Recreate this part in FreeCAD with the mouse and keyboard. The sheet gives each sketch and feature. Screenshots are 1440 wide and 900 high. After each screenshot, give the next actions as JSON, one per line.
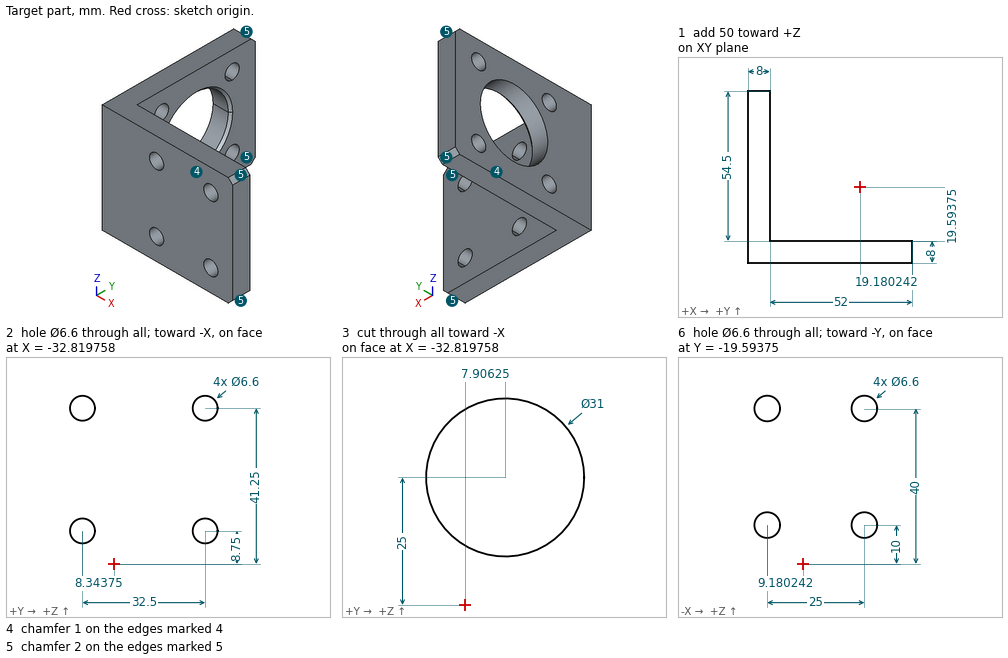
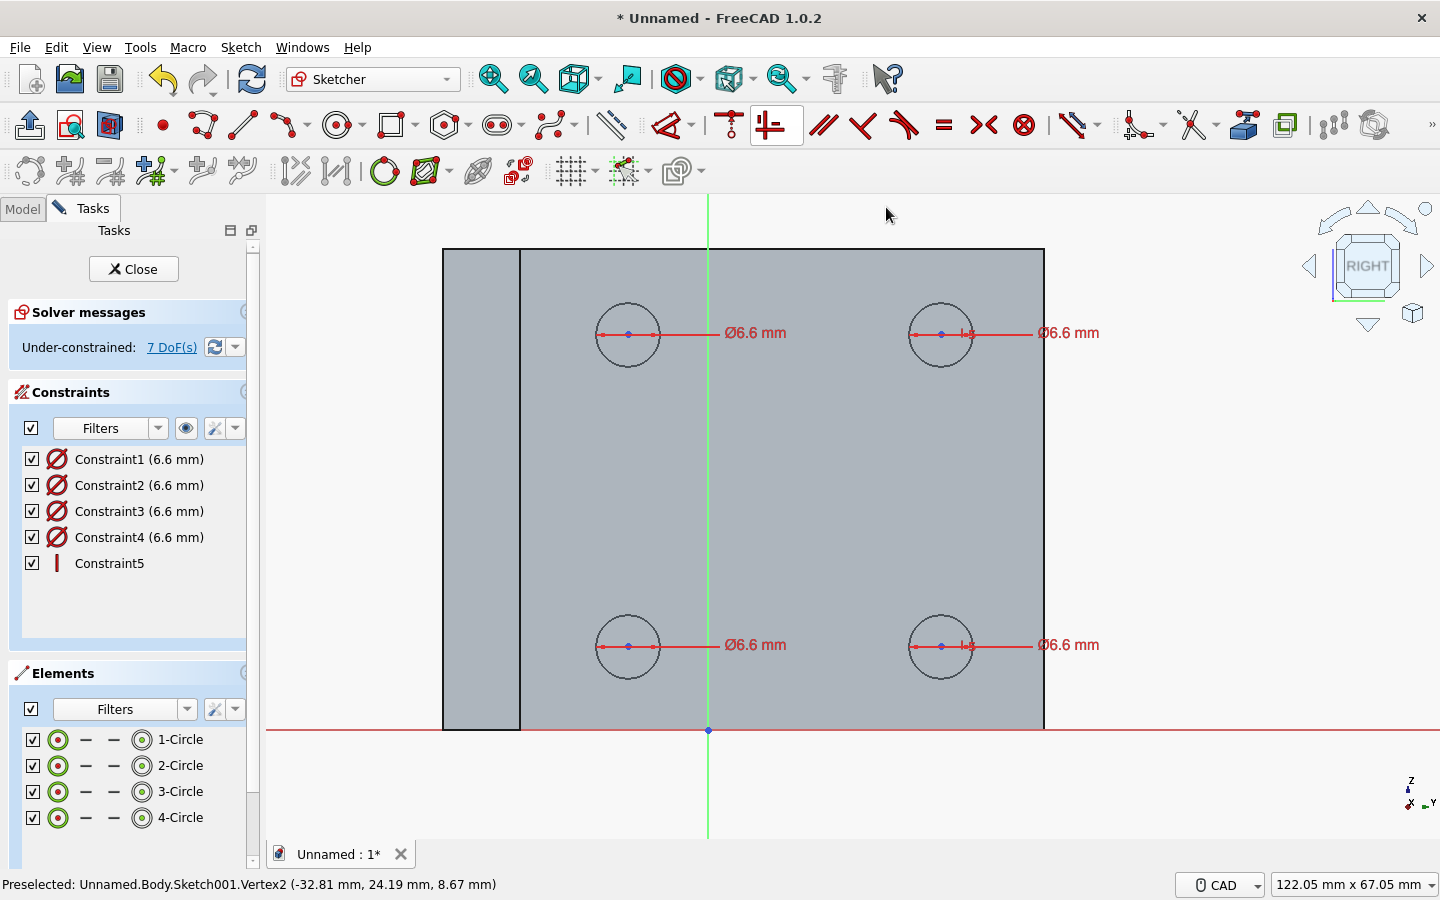
{"action": "left_click", "coordinate": [941, 647]}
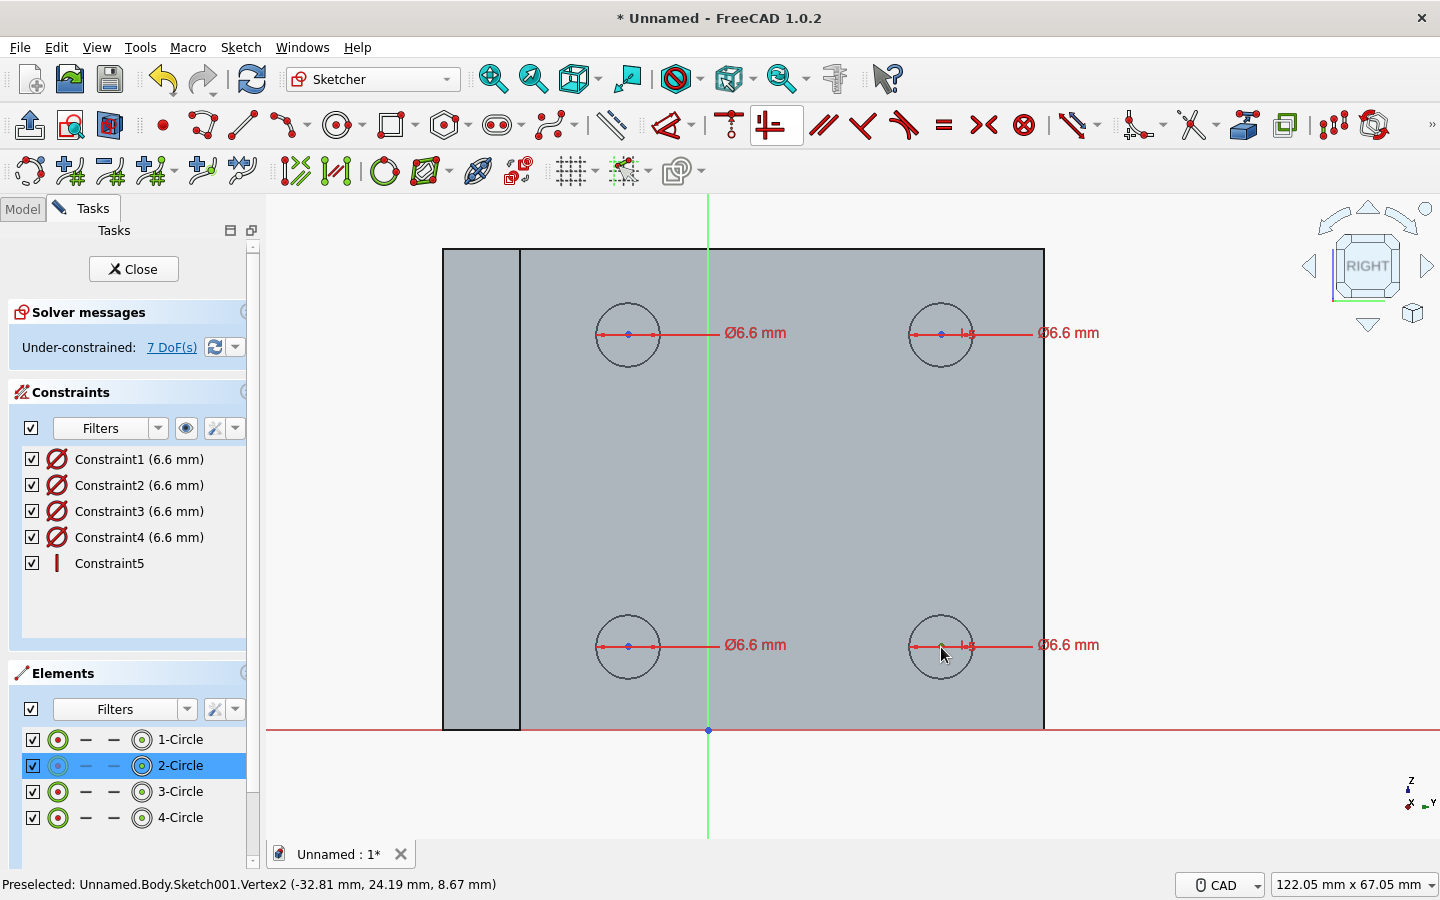
{"action": "left_click", "coordinate": [628, 647]}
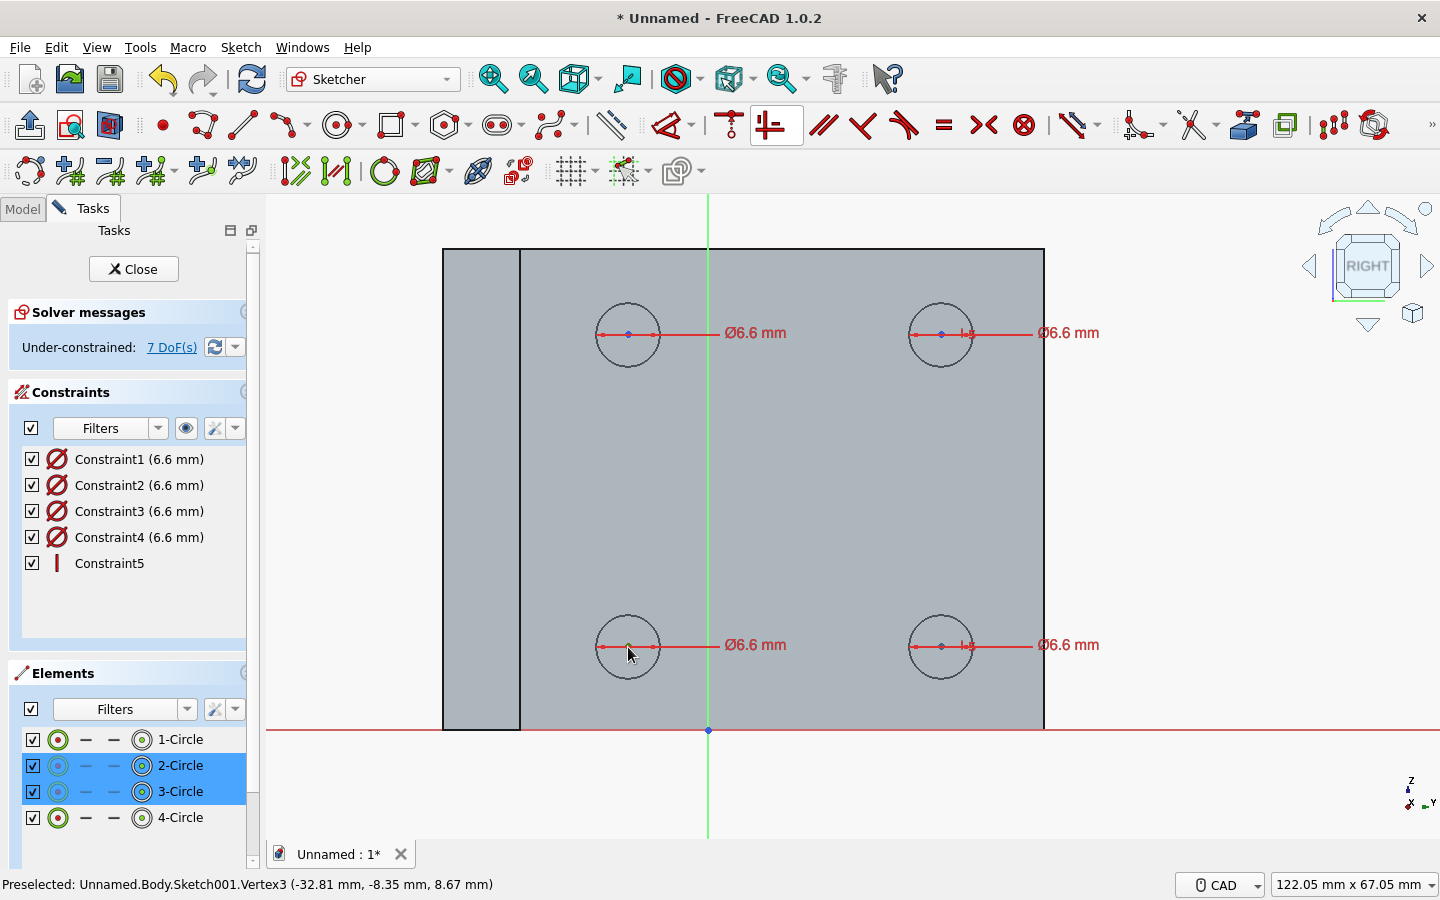
{"action": "key", "text": "h"}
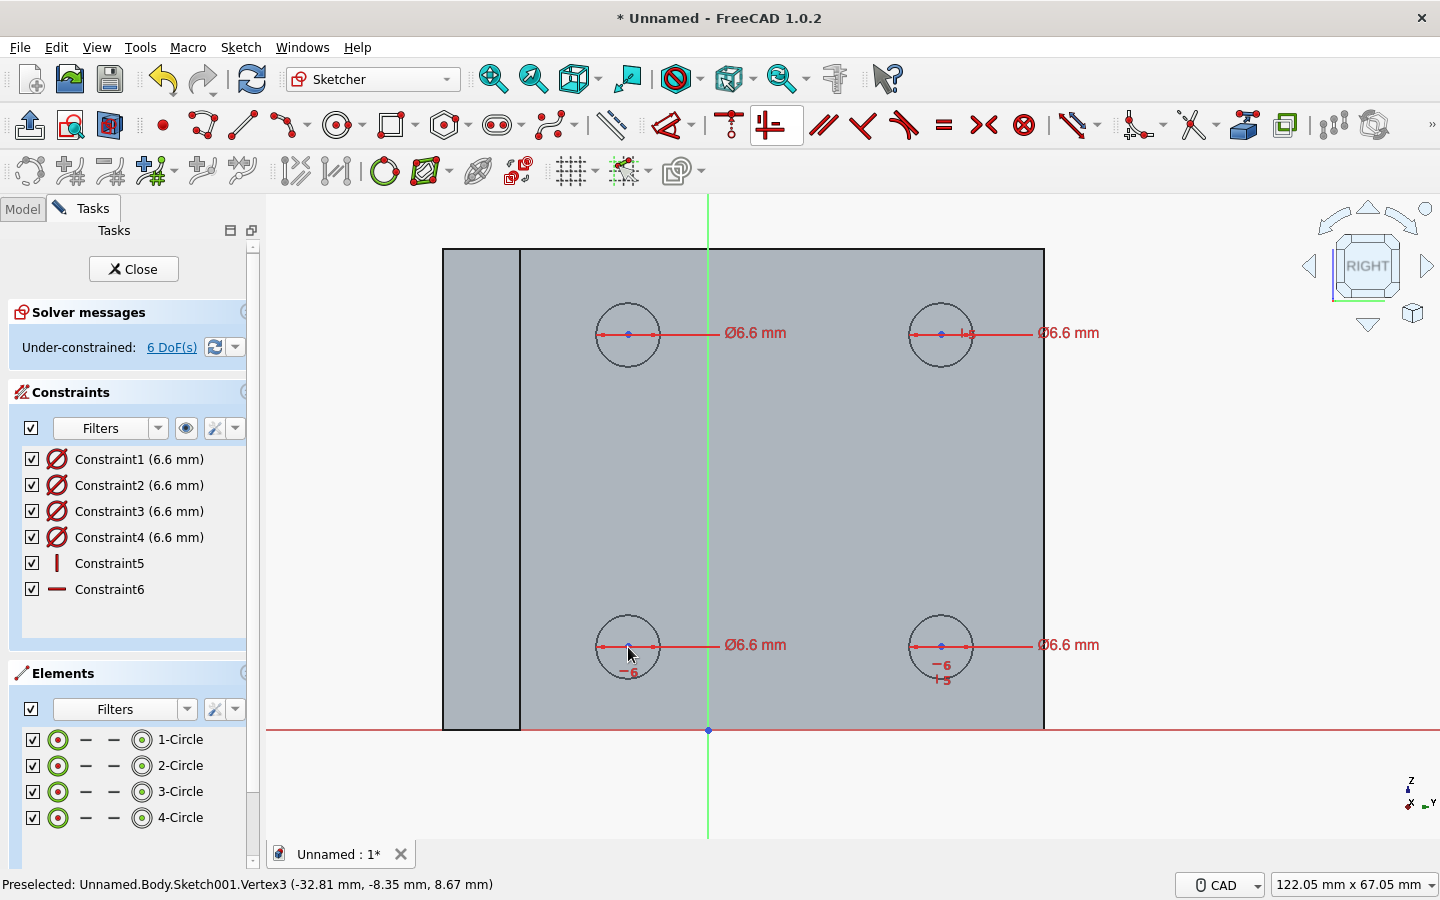
{"action": "left_click", "coordinate": [628, 647]}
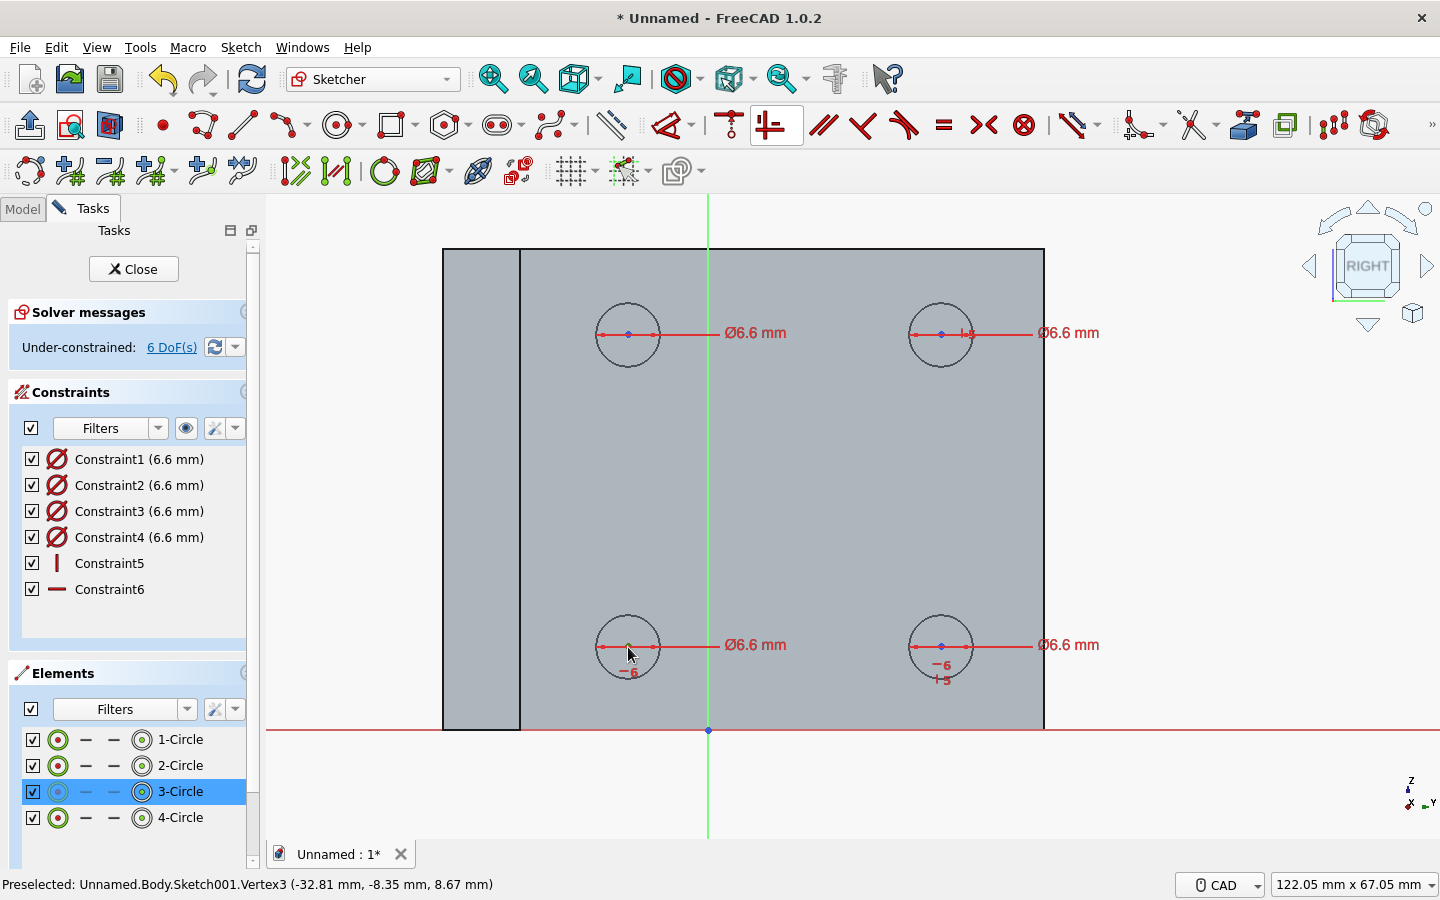
{"action": "left_click", "coordinate": [628, 335]}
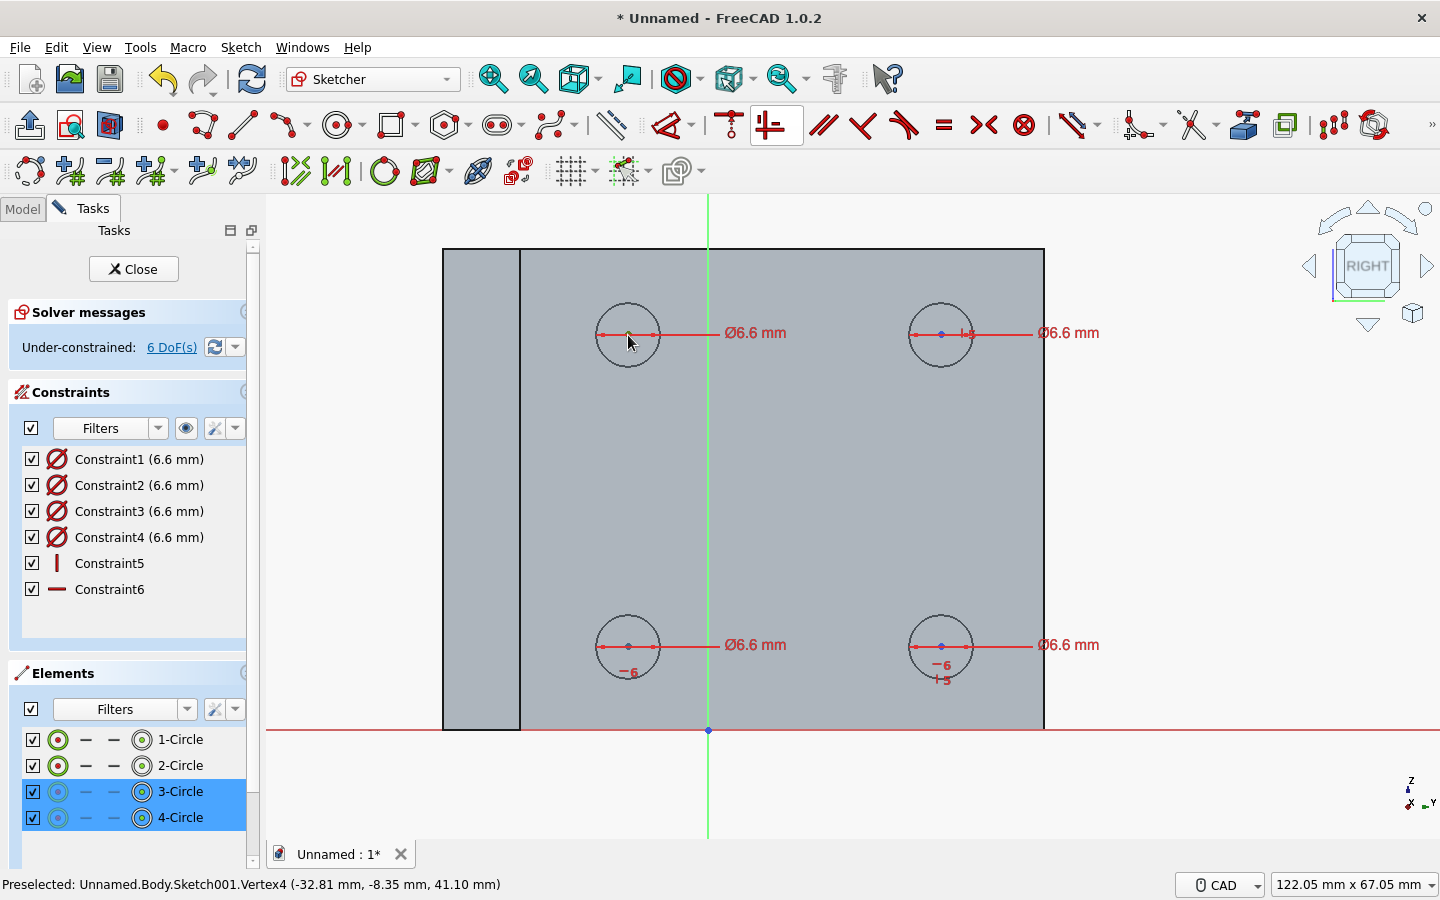
{"action": "left_click", "coordinate": [798, 126]}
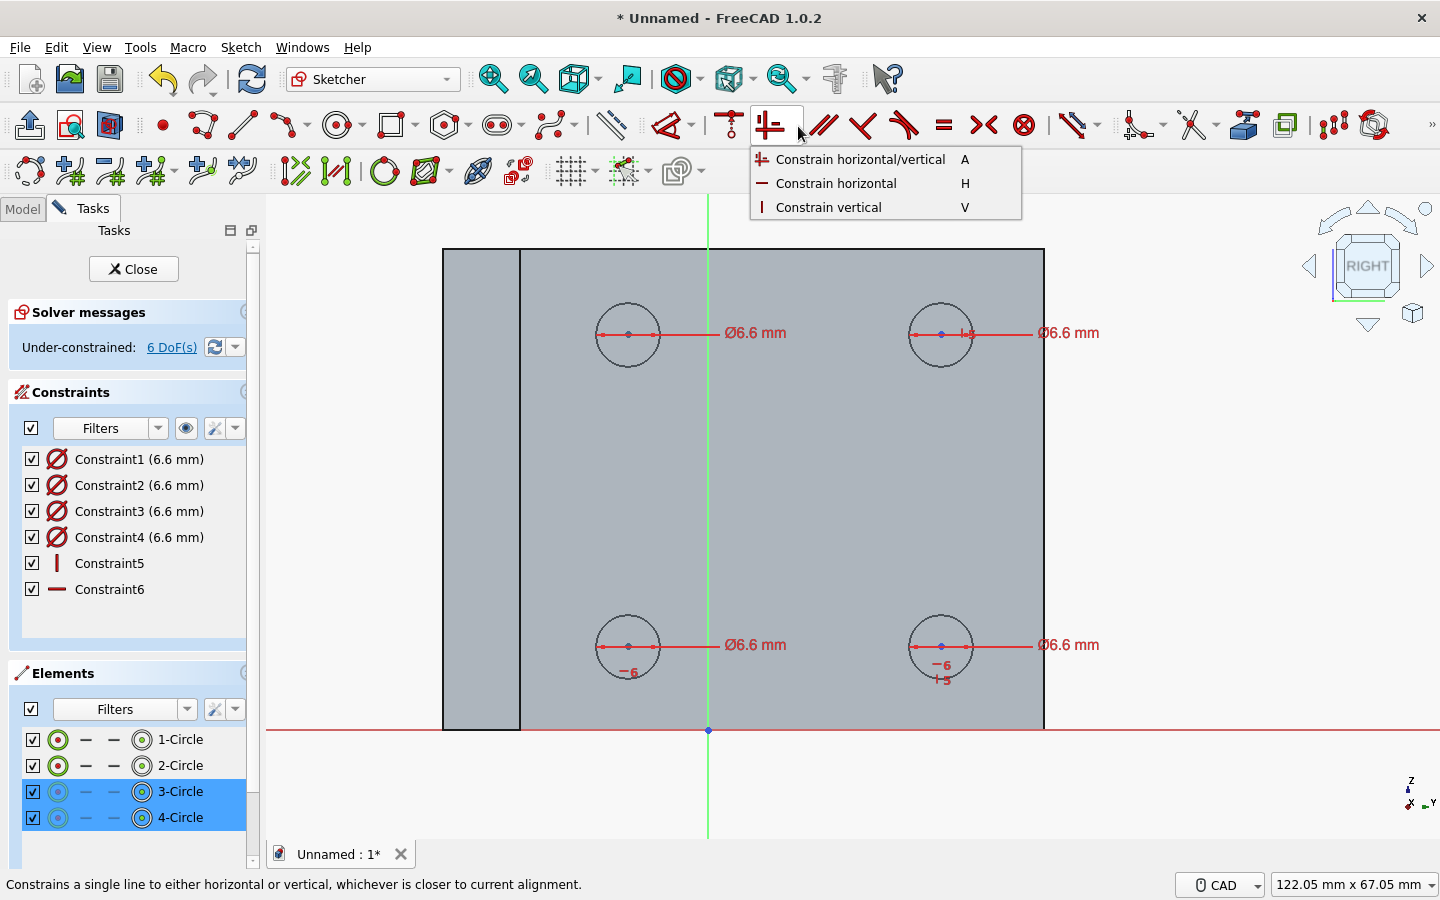
{"action": "left_click", "coordinate": [886, 207]}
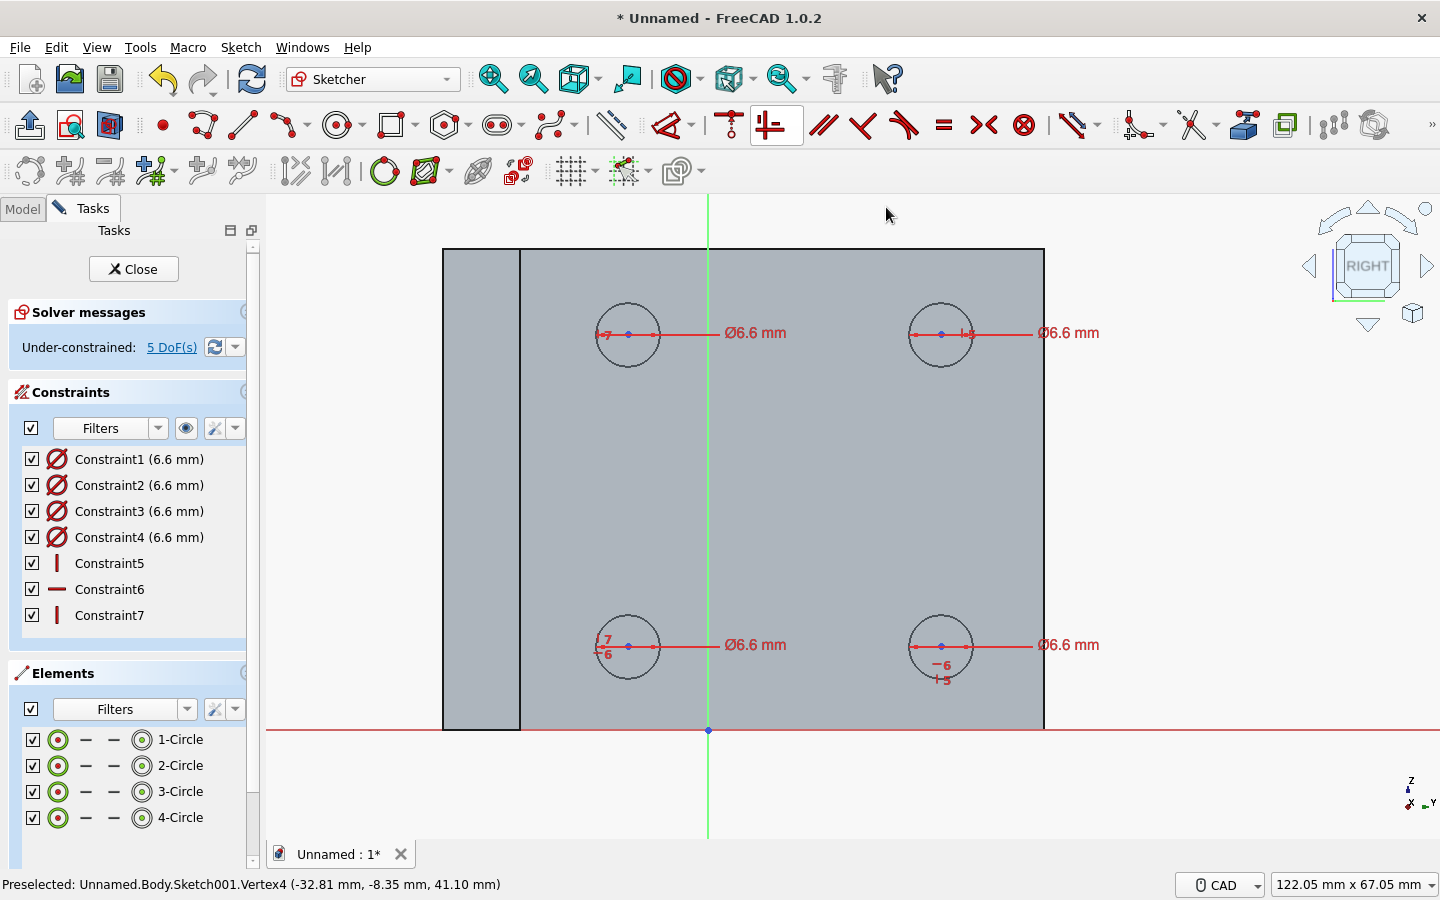
{"action": "left_click", "coordinate": [941, 335]}